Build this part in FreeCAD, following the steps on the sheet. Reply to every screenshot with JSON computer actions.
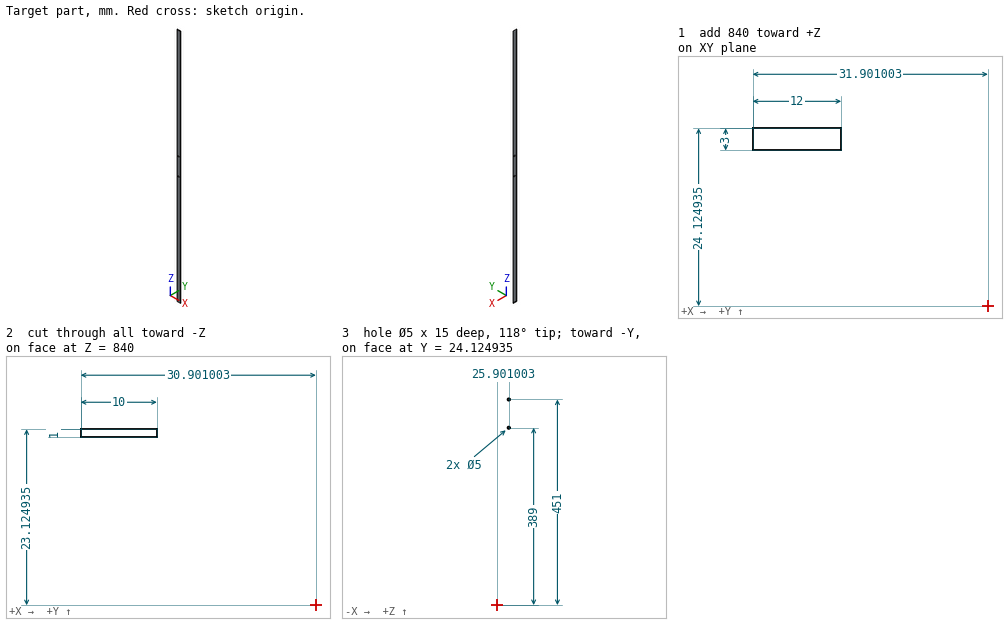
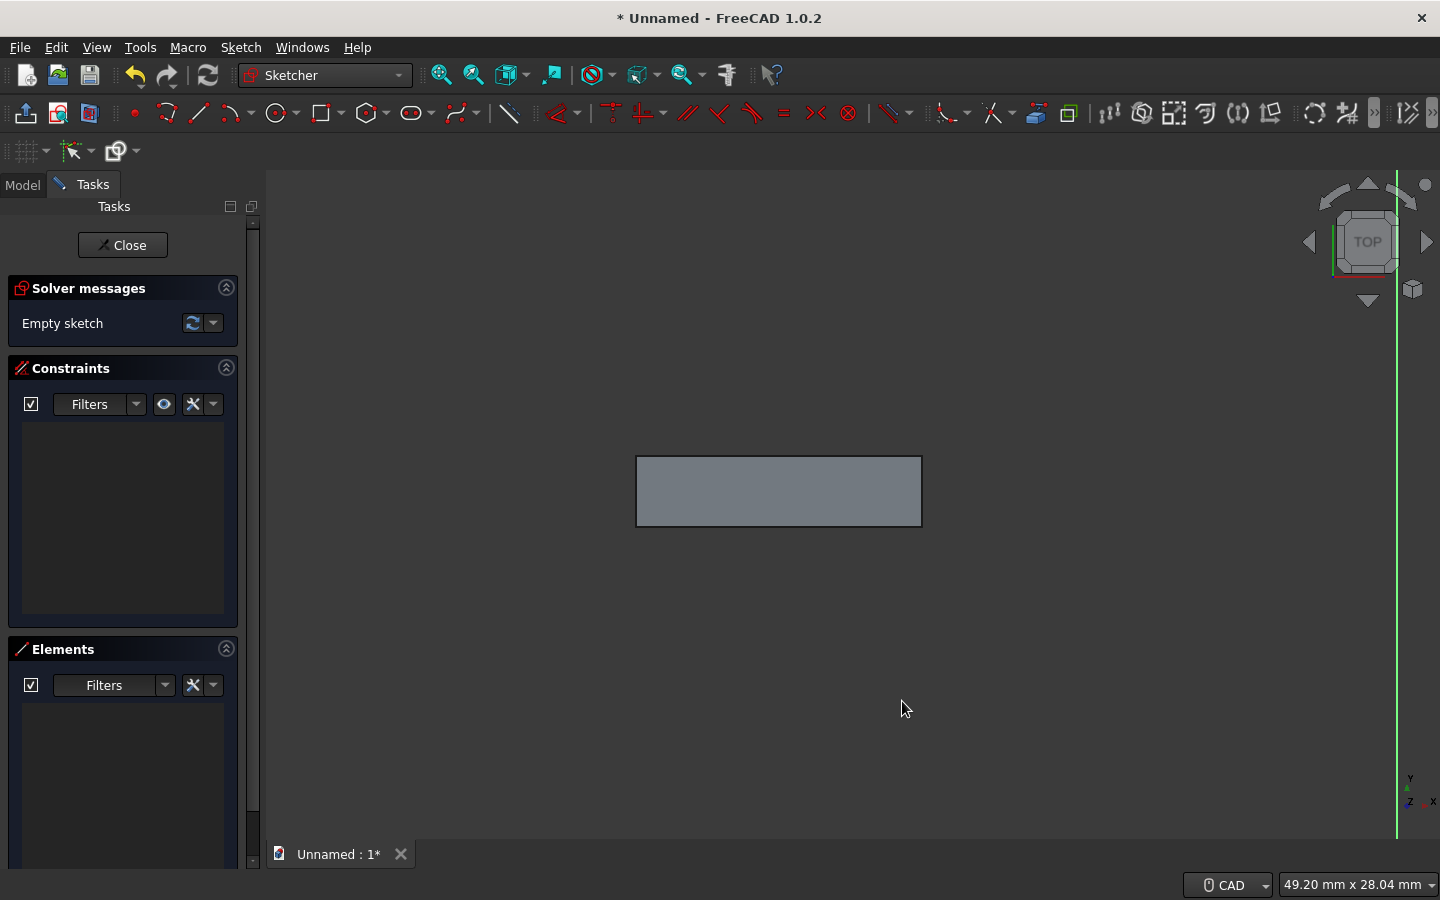
{"action": "scroll", "coordinate": [776, 484], "scroll_direction": "up", "scroll_amount": 5}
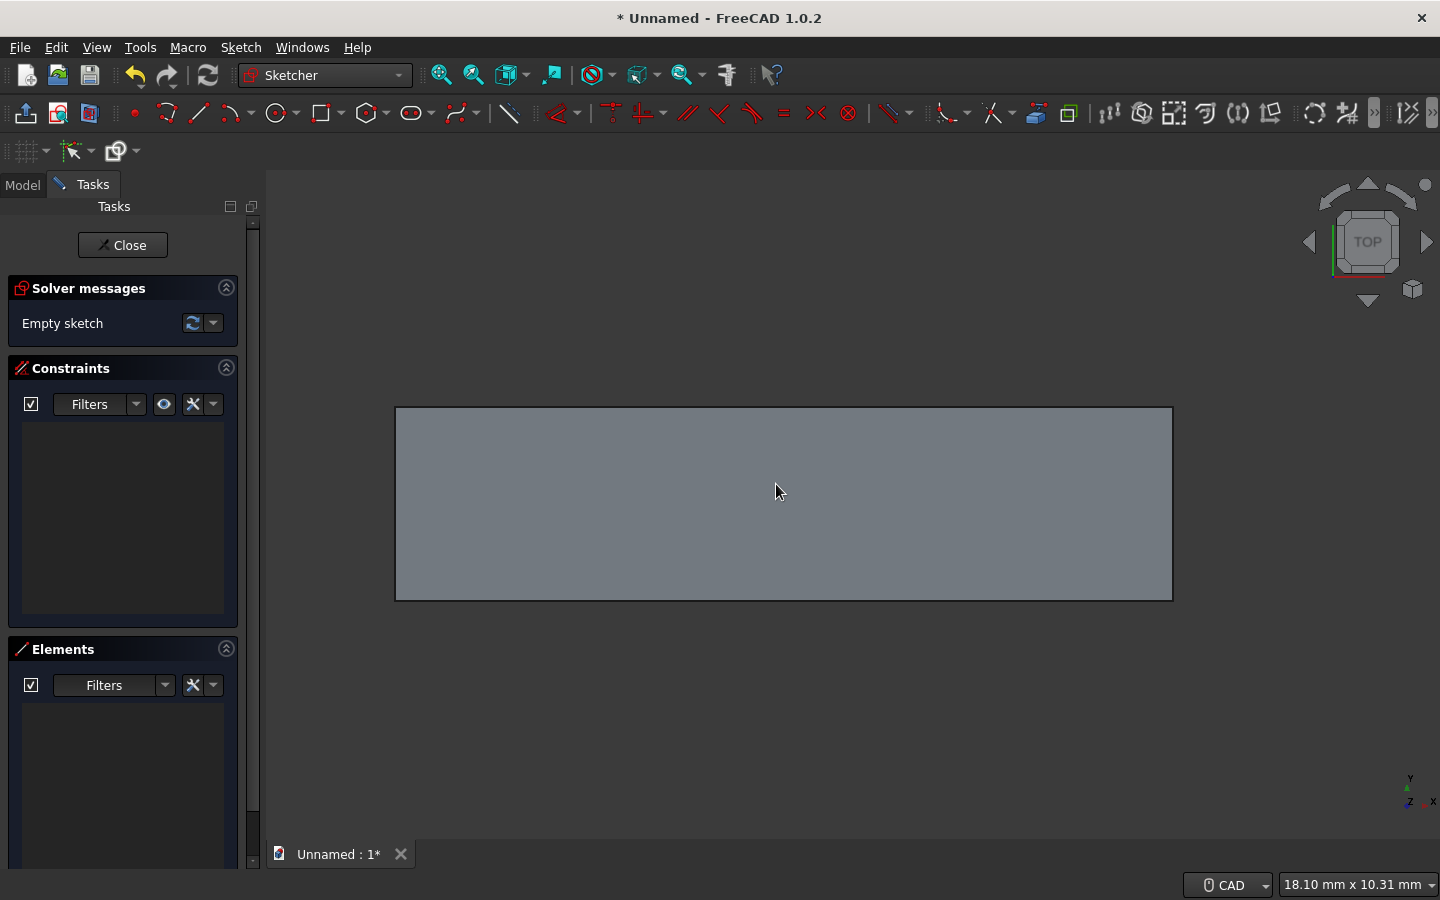
{"action": "left_click", "coordinate": [322, 114]}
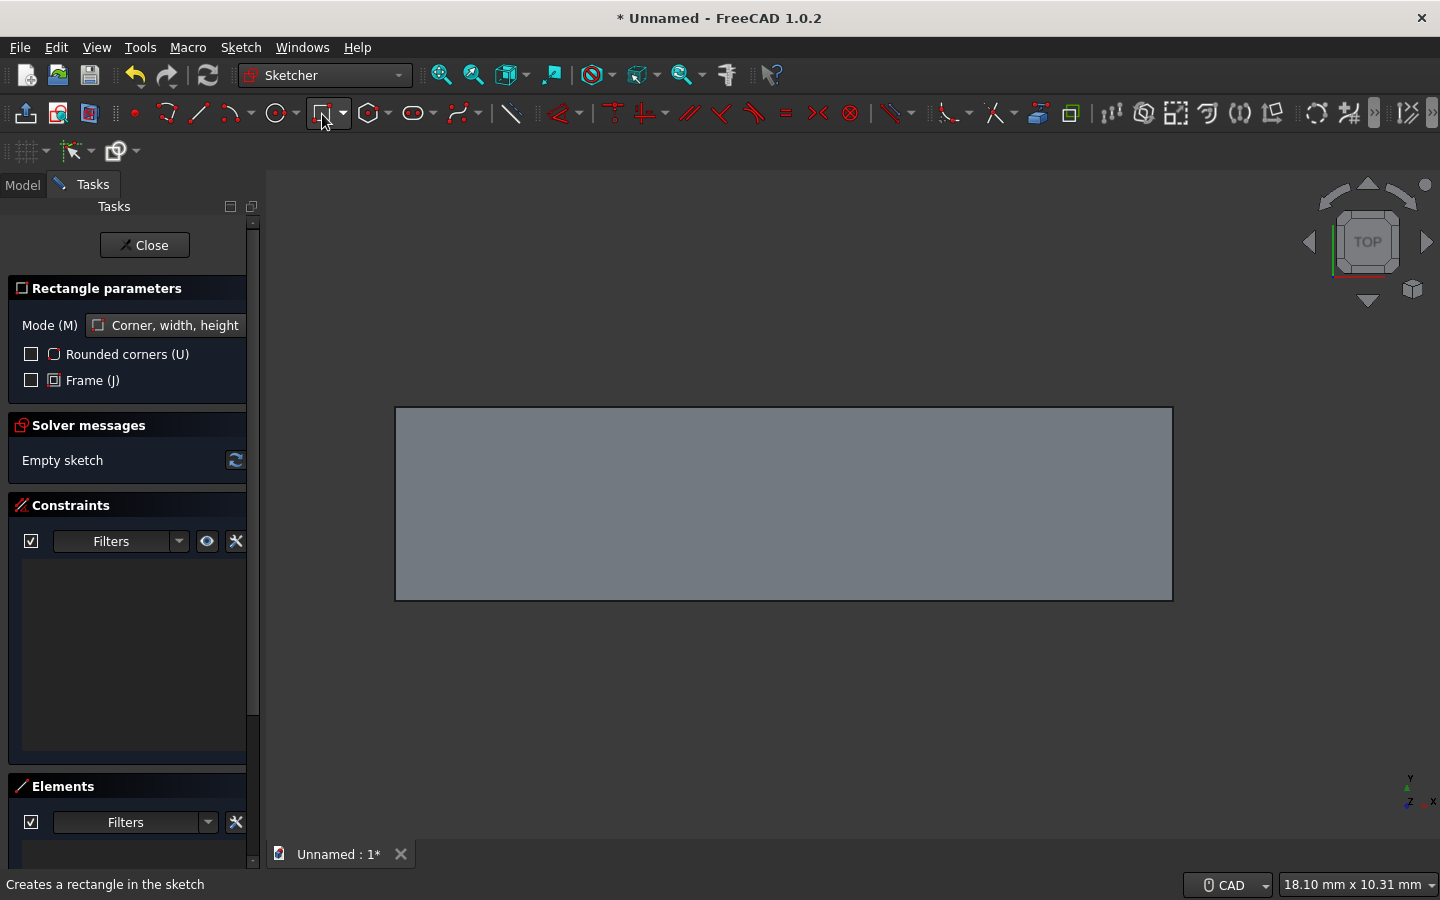
{"action": "left_click", "coordinate": [460, 471]}
{"action": "mouse_move", "coordinate": [1108, 536]}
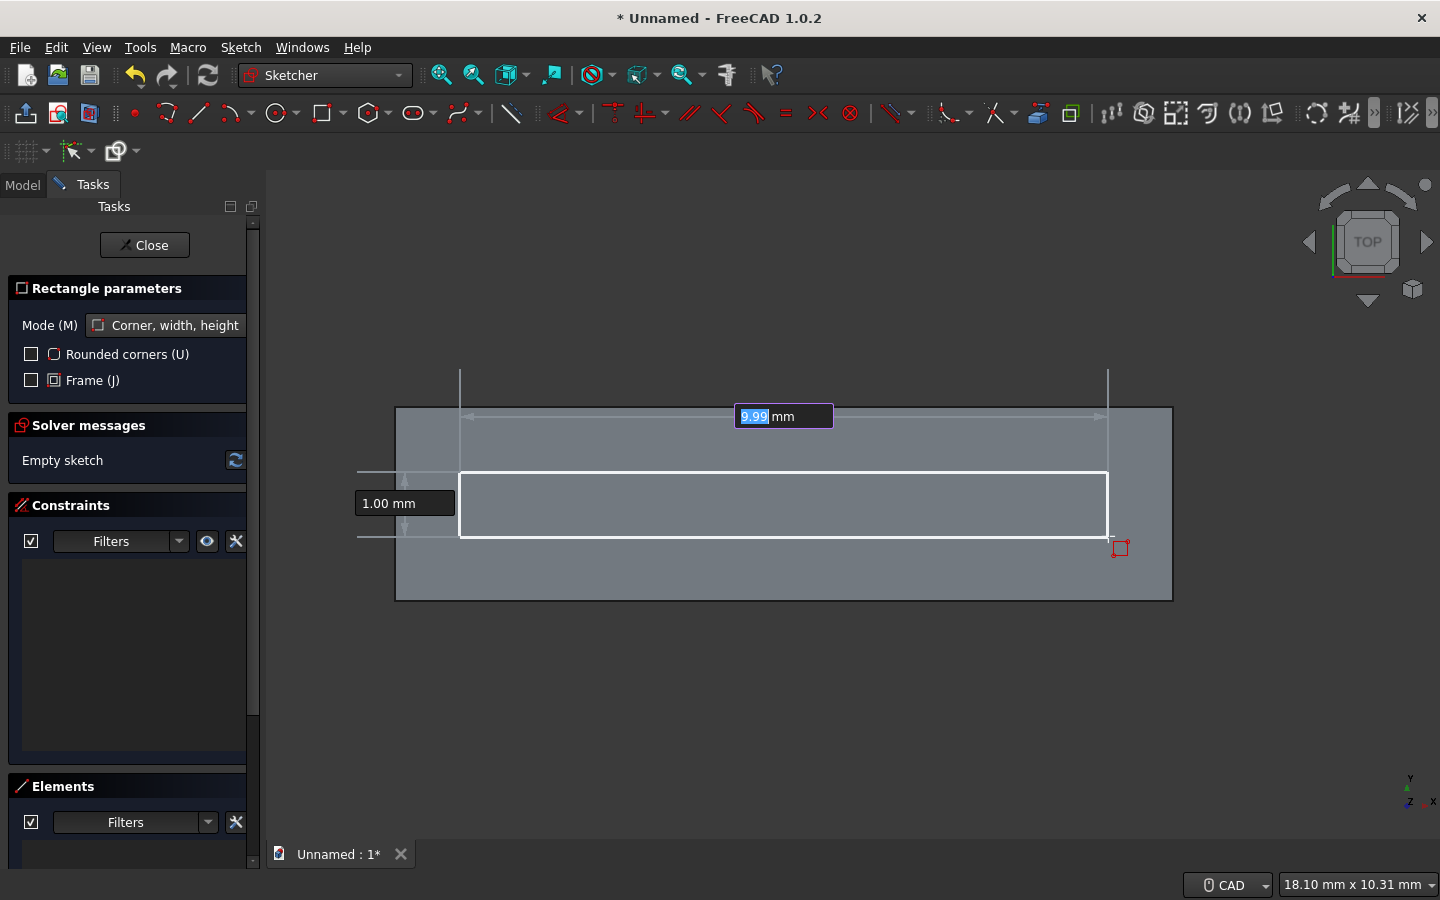
{"action": "type", "text": "10"}
{"action": "key", "text": "Tab"}
{"action": "type", "text": "1"}
{"action": "key", "text": "Return"}
{"action": "key", "text": "Escape"}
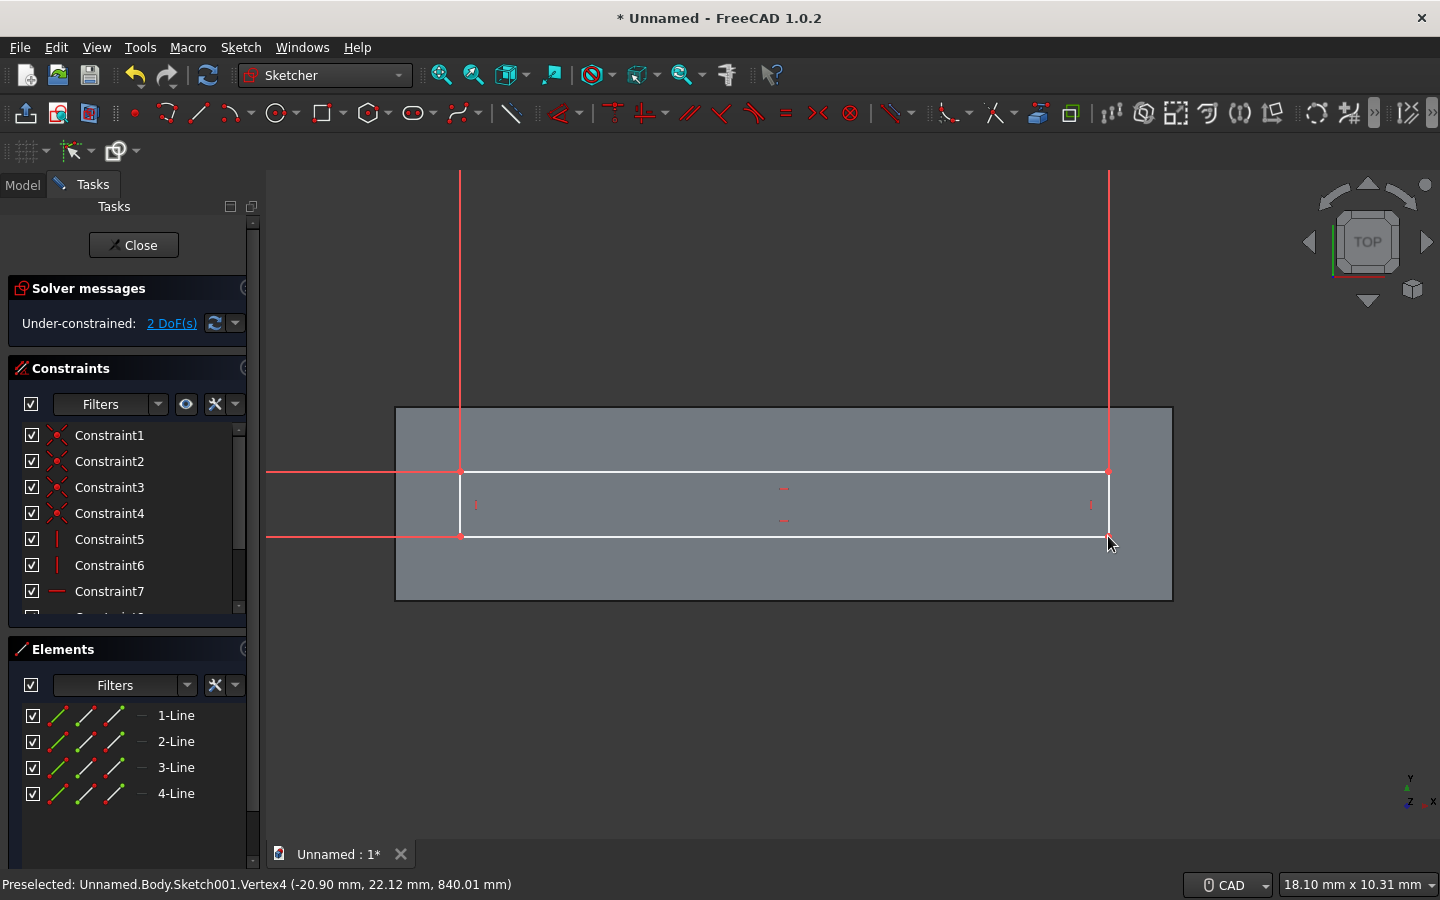
{"action": "left_click", "coordinate": [558, 114]}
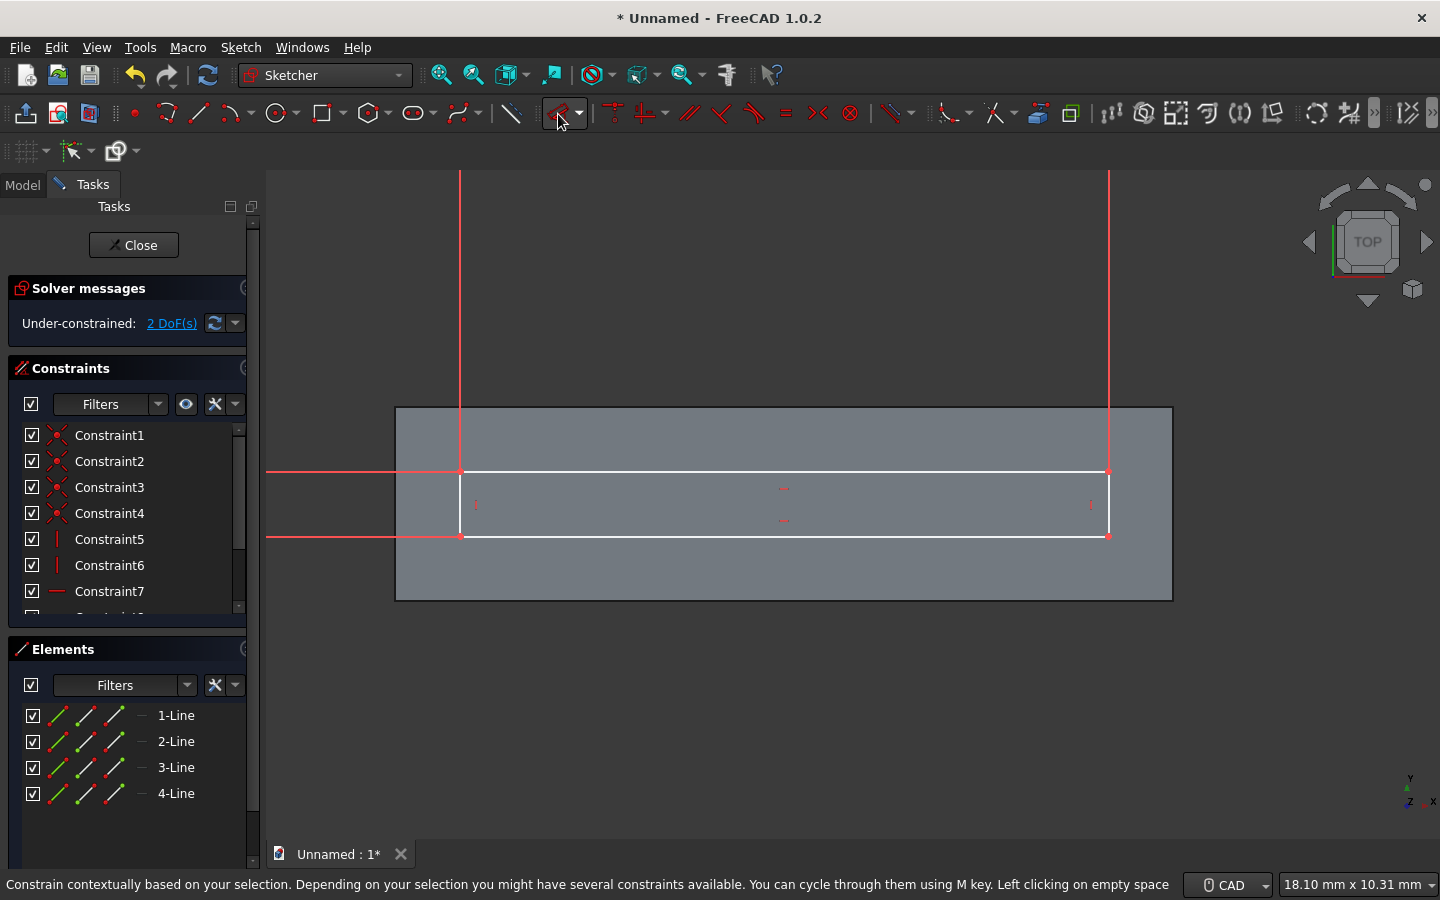
{"action": "left_click", "coordinate": [460, 472]}
{"action": "left_click", "coordinate": [867, 438]}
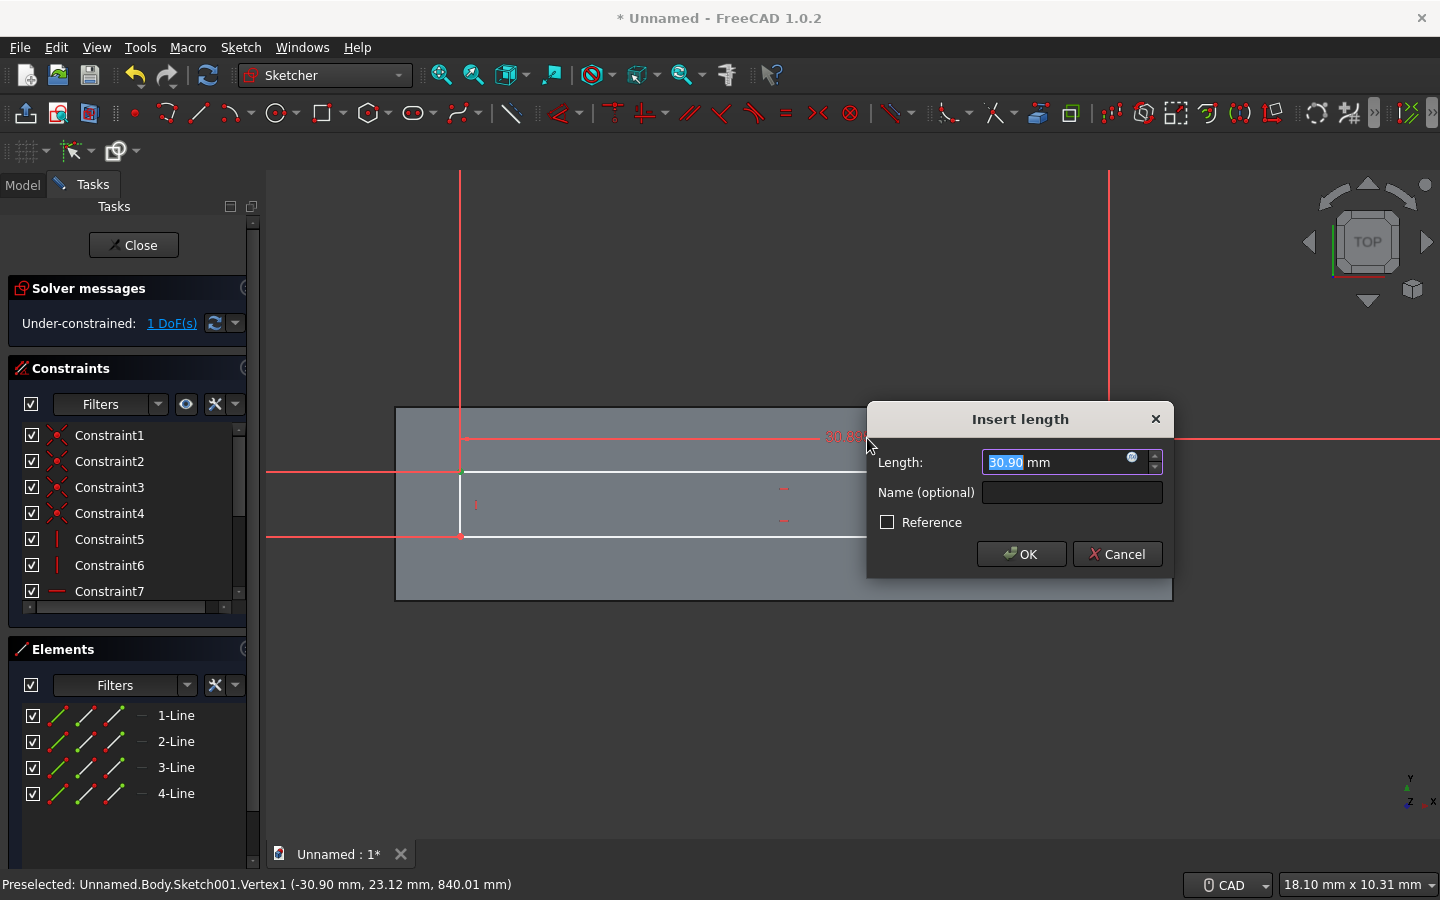
{"action": "type", "text": "30.901003"}
{"action": "key", "text": "Return"}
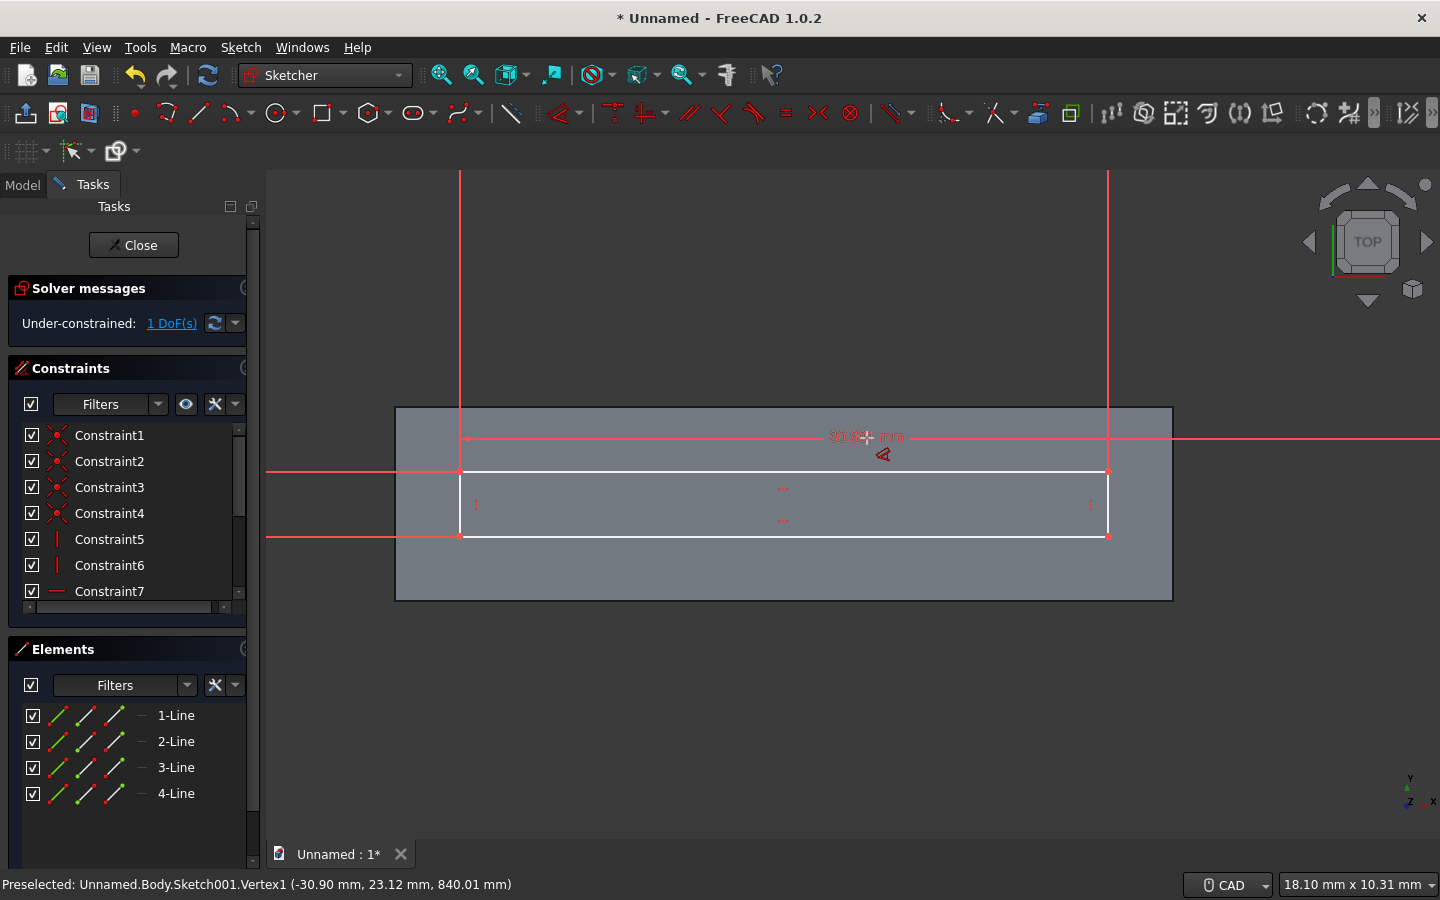
{"action": "left_click", "coordinate": [460, 472]}
{"action": "left_click", "coordinate": [426, 641]}